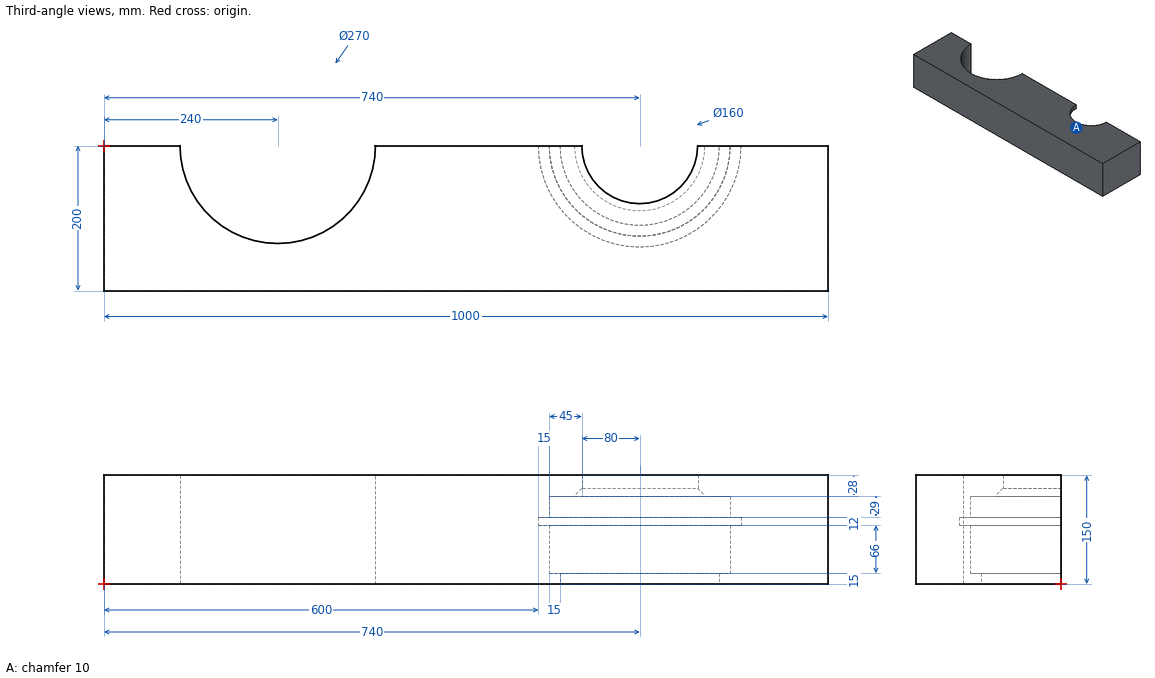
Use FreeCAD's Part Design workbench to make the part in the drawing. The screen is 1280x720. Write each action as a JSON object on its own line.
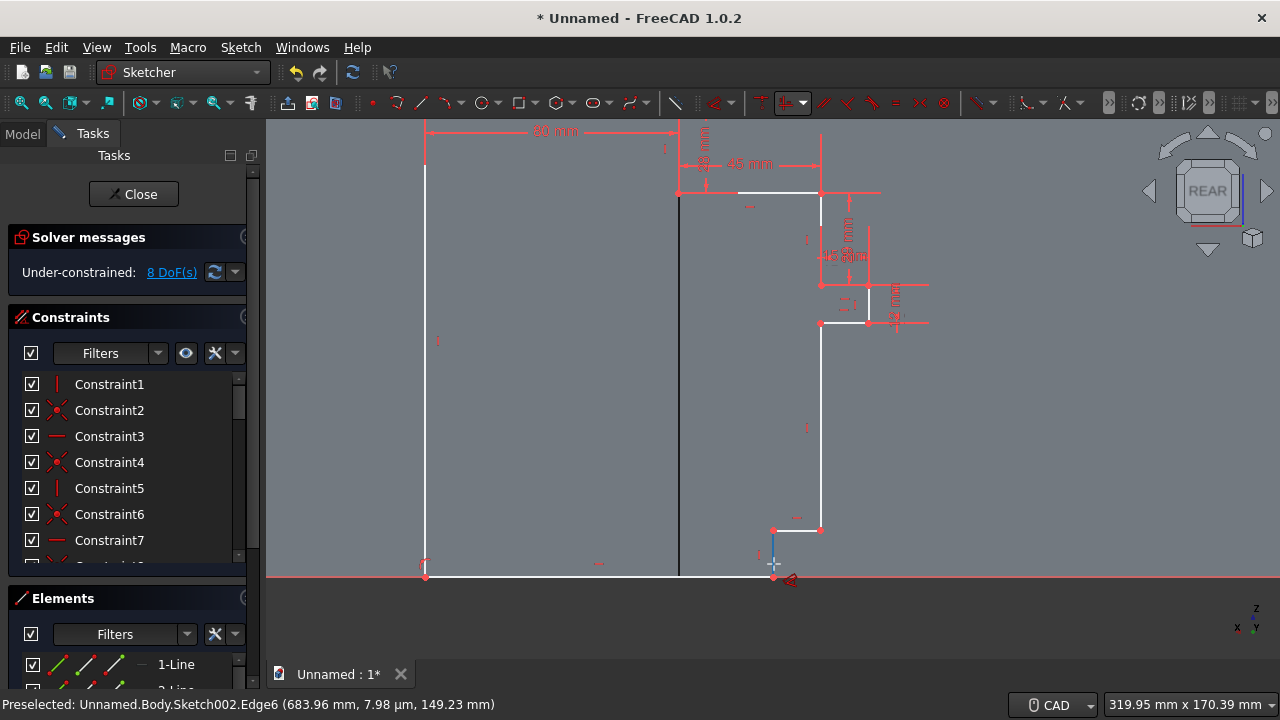
{"action": "left_click", "coordinate": [773, 563]}
{"action": "left_click", "coordinate": [807, 554]}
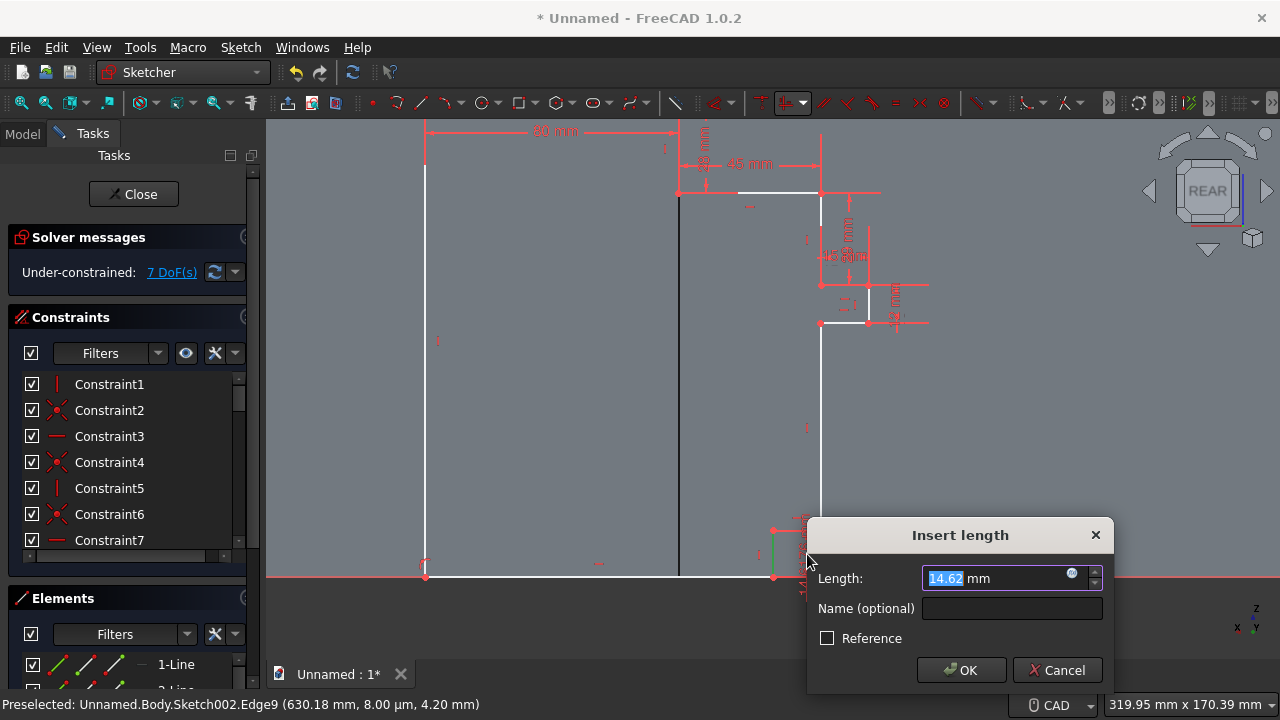
{"action": "type", "text": "15"}
{"action": "key", "text": "Return"}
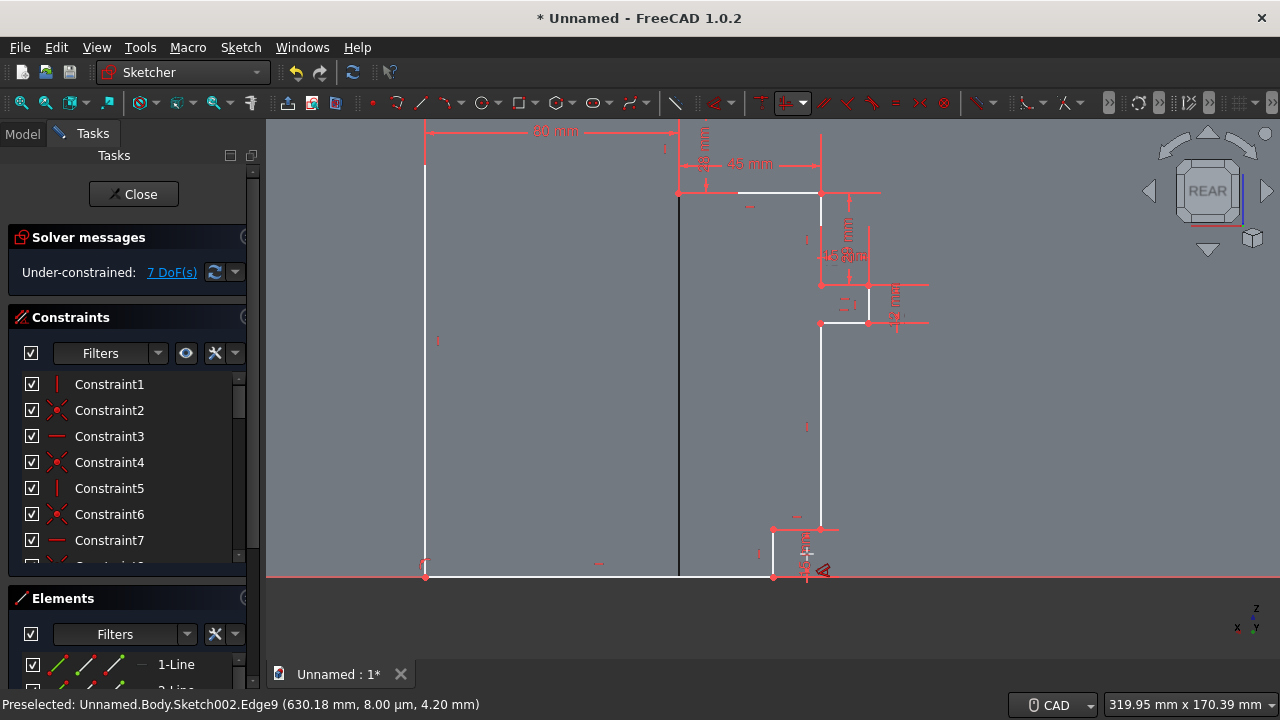
{"action": "left_click", "coordinate": [788, 530]}
{"action": "left_click", "coordinate": [797, 496]}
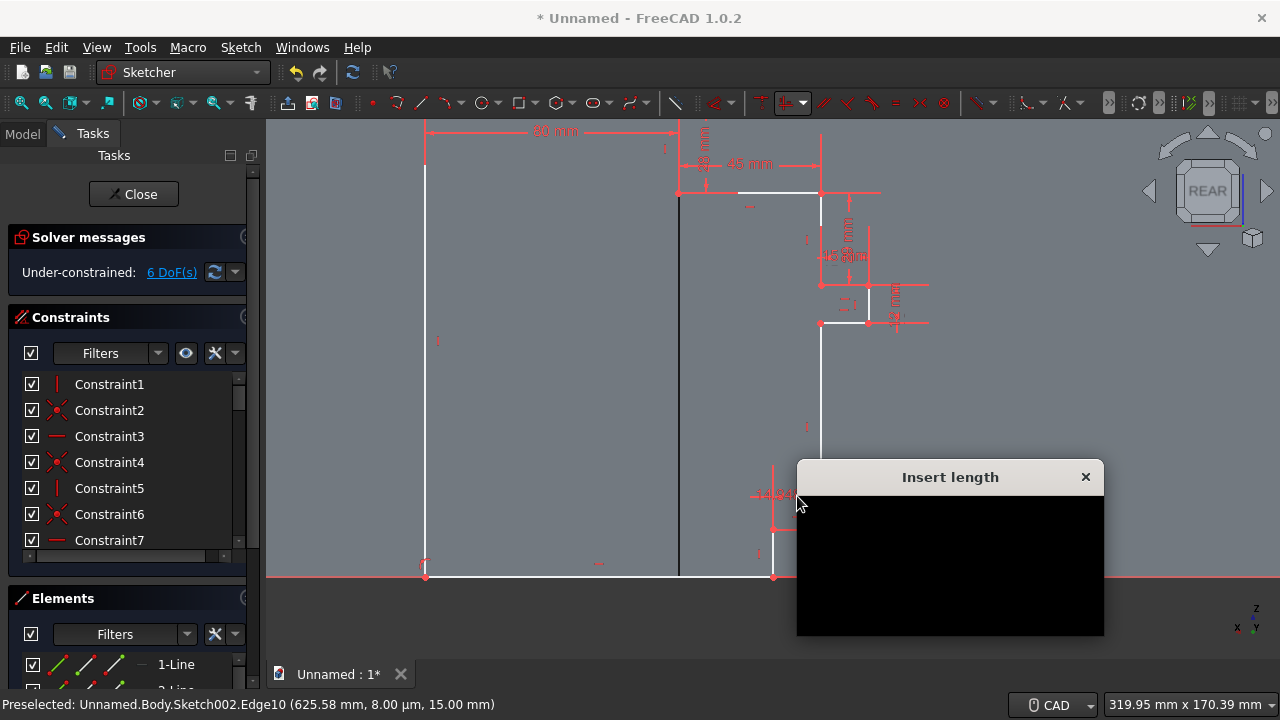
{"action": "type", "text": "15"}
{"action": "key", "text": "Return"}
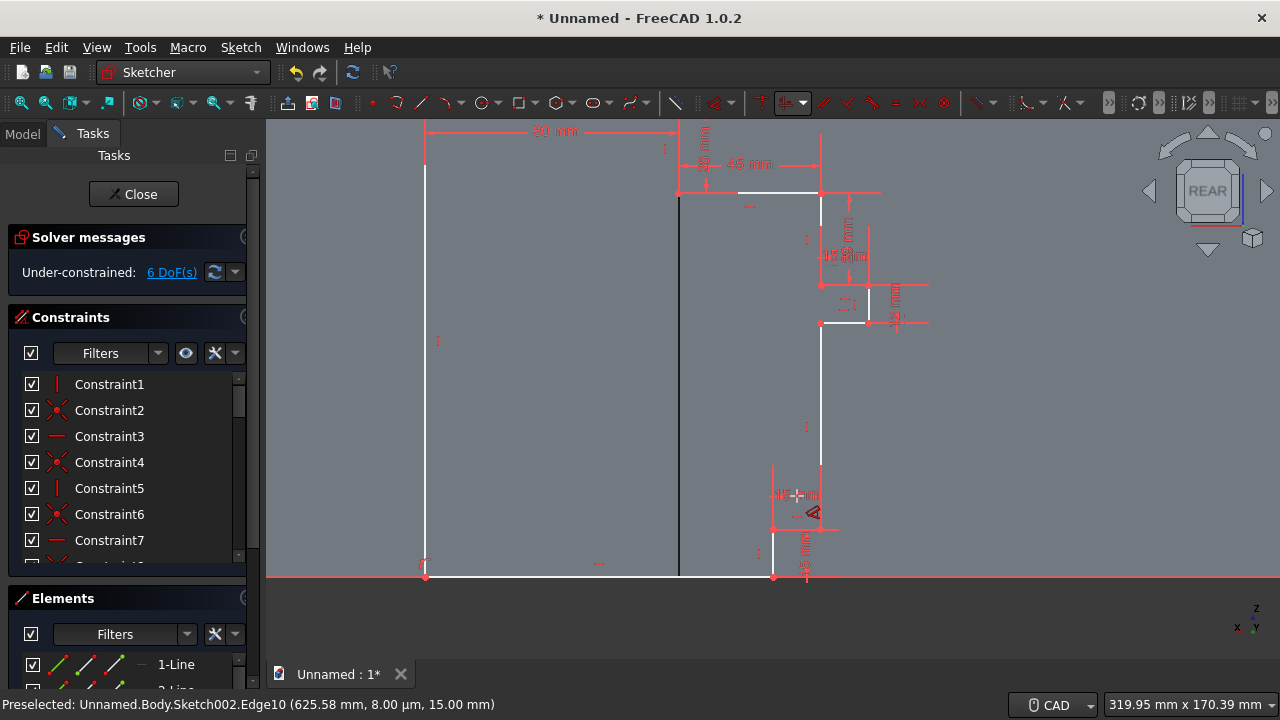
{"action": "left_click", "coordinate": [821, 468]}
{"action": "left_click", "coordinate": [855, 426]}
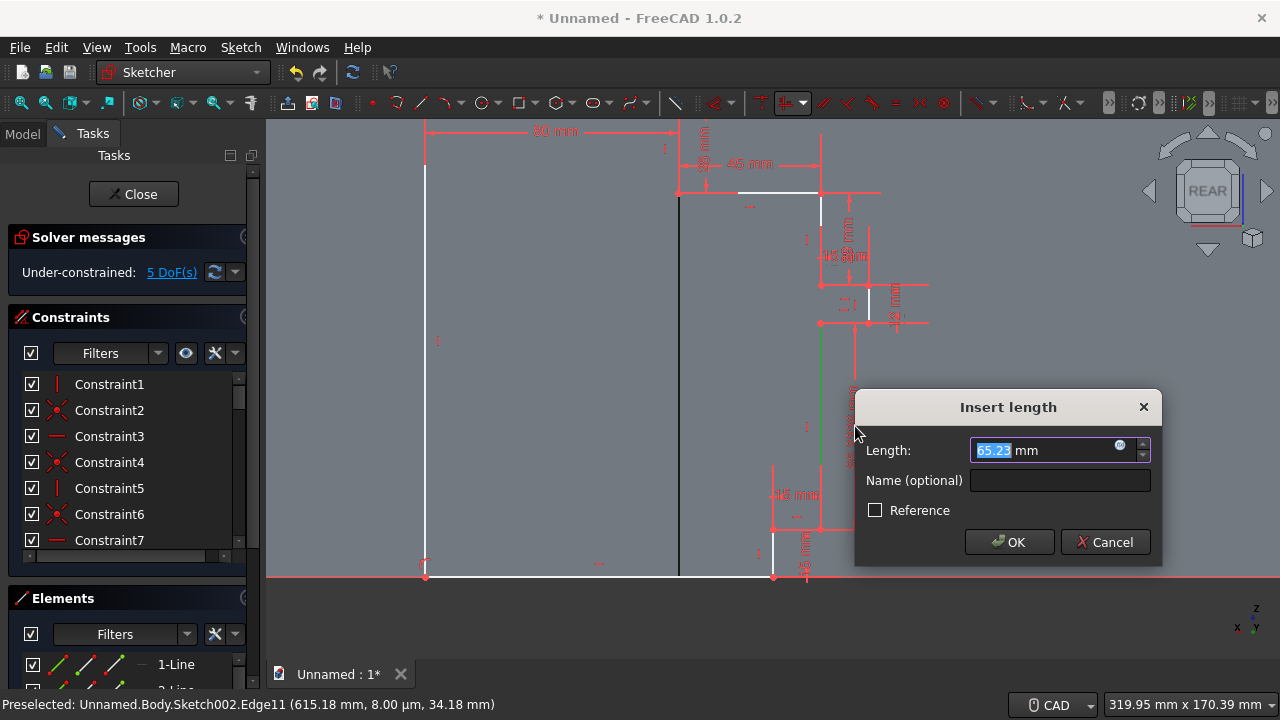
{"action": "type", "text": "66"}
{"action": "key", "text": "Return"}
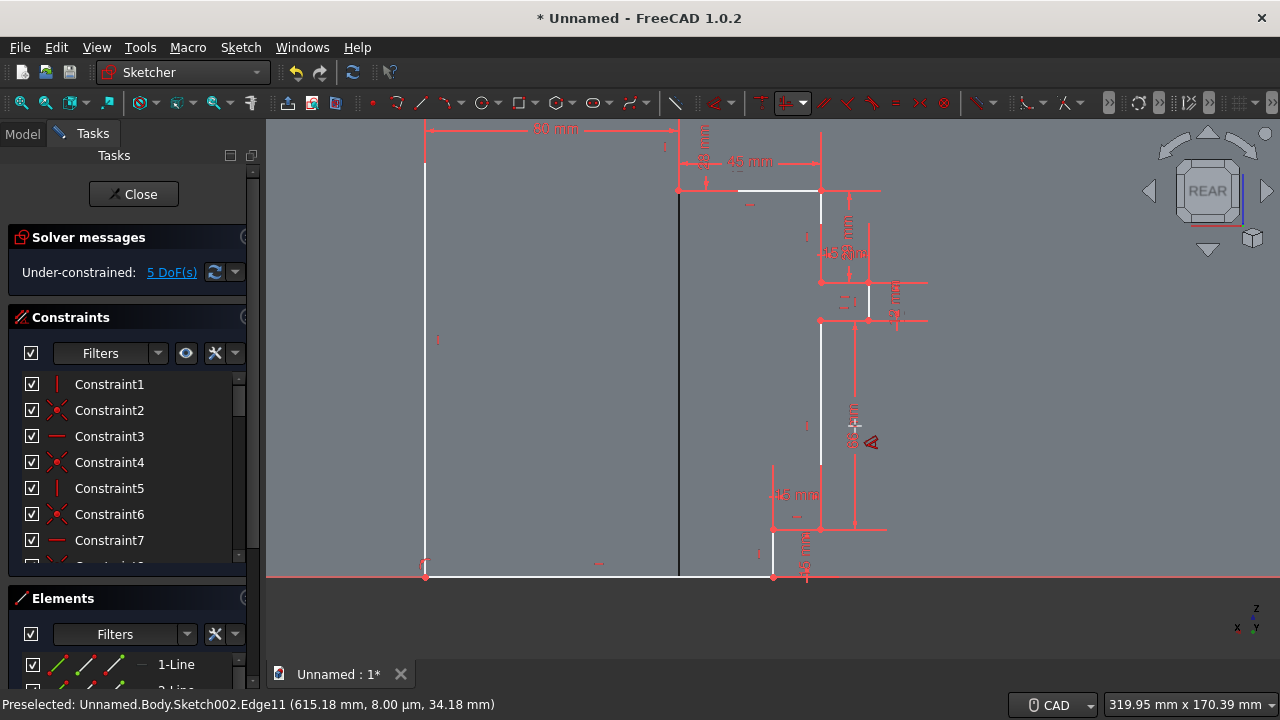
{"action": "left_click", "coordinate": [835, 321]}
{"action": "left_click", "coordinate": [845, 355]}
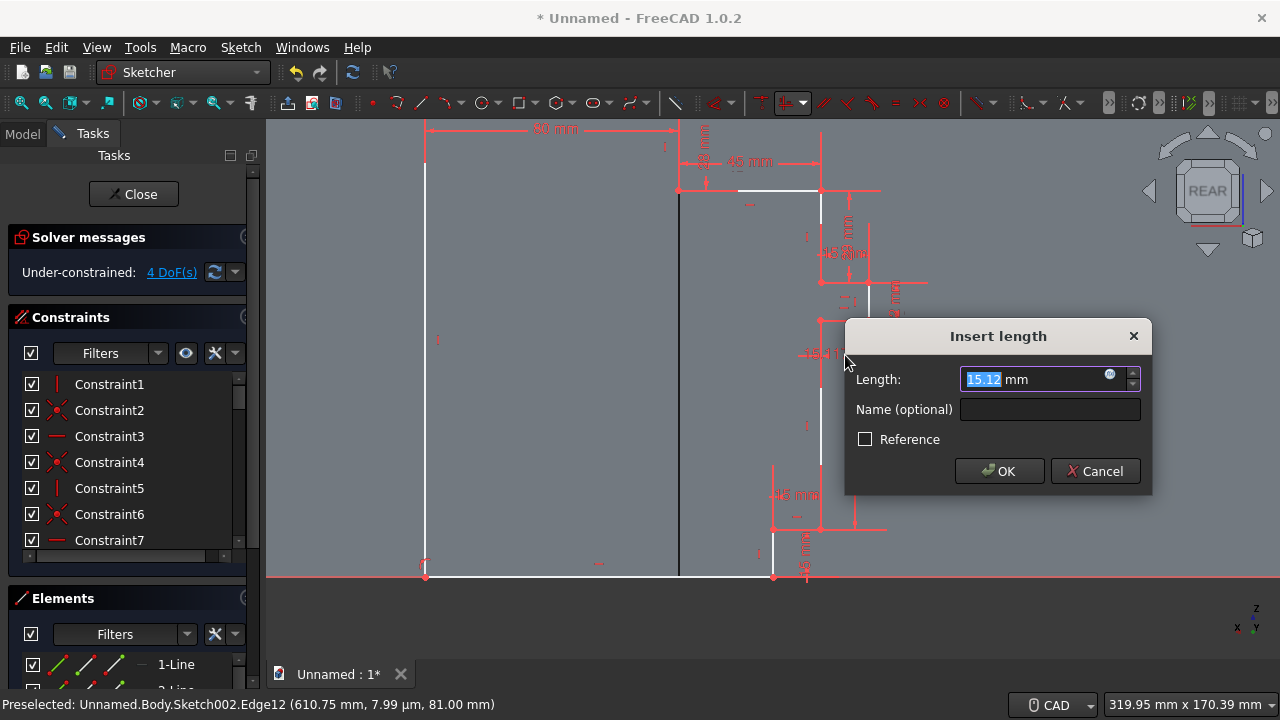
{"action": "type", "text": "15"}
{"action": "key", "text": "Return"}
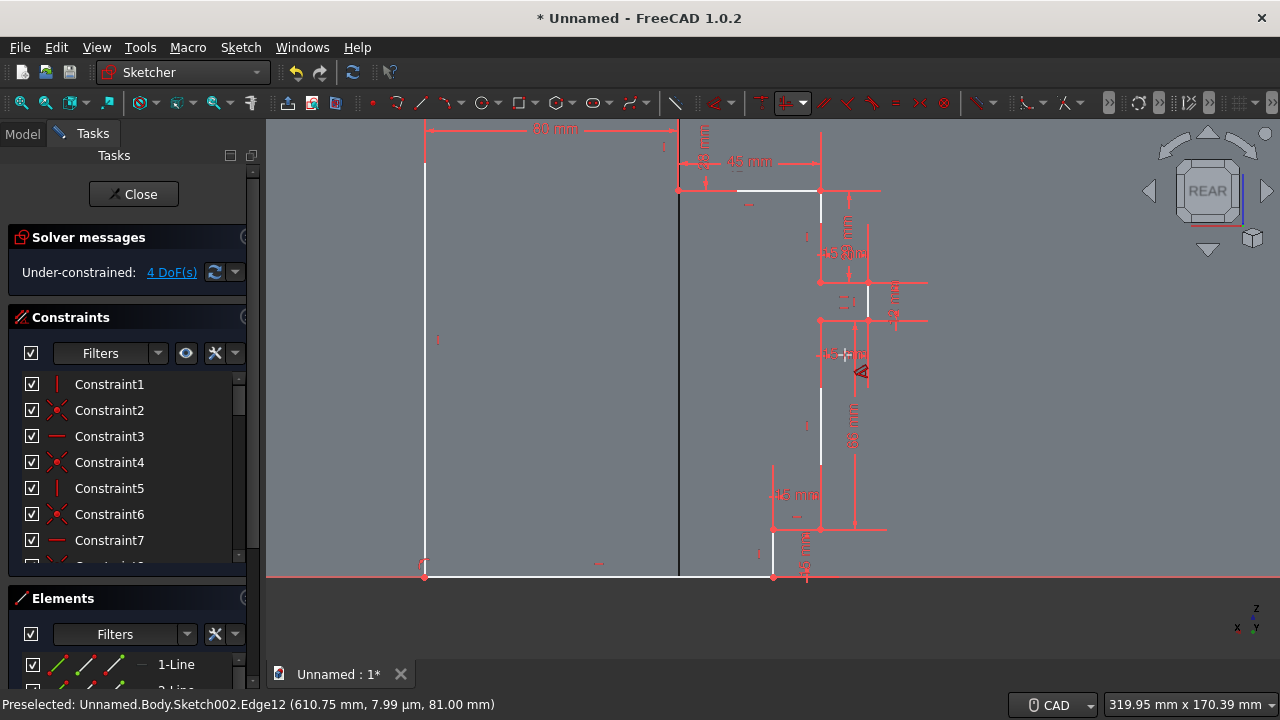
{"action": "left_click", "coordinate": [868, 321]}
{"action": "left_click", "coordinate": [992, 611]}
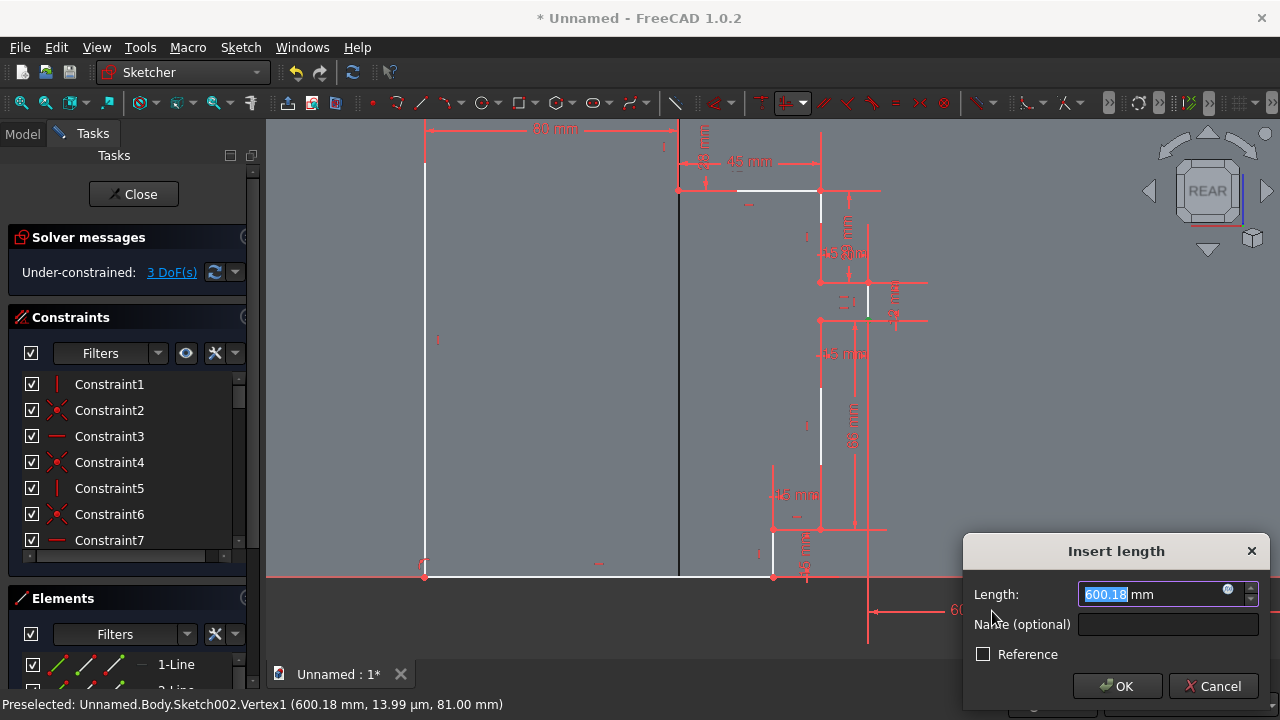
{"action": "type", "text": "600"}
{"action": "key", "text": "Return"}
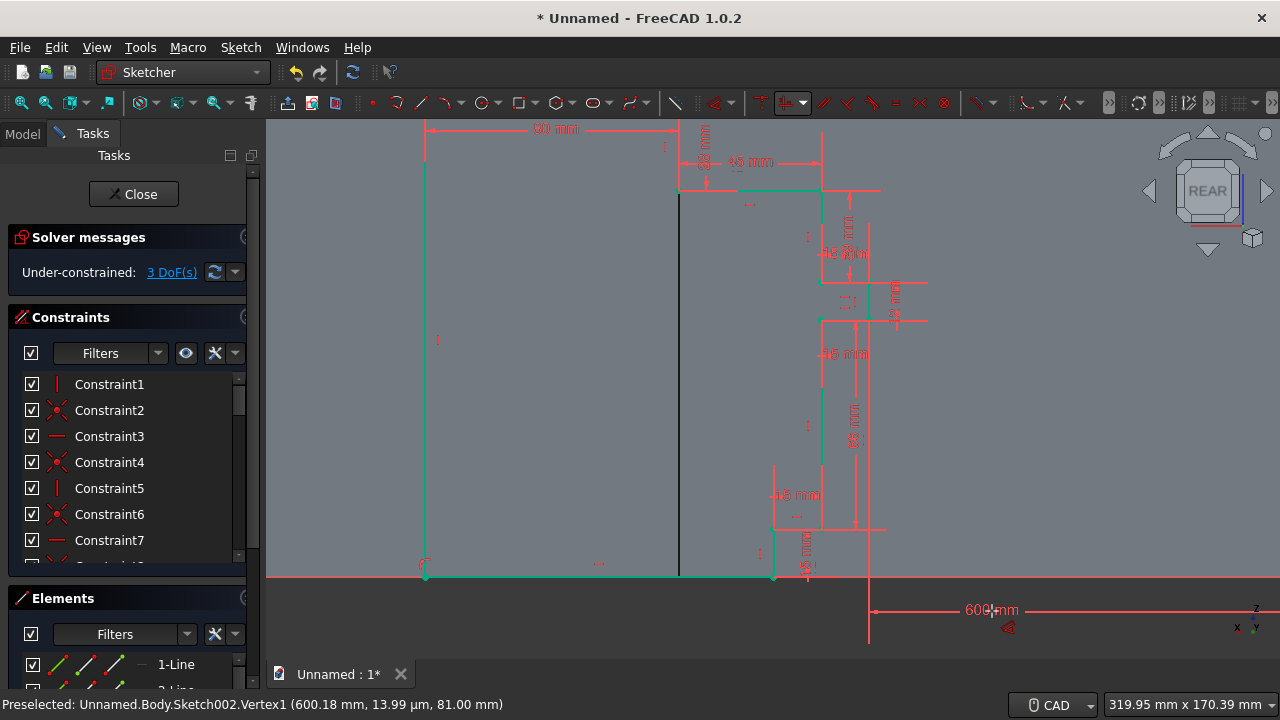
{"action": "scroll", "coordinate": [774, 565], "scroll_direction": "down", "scroll_amount": 3}